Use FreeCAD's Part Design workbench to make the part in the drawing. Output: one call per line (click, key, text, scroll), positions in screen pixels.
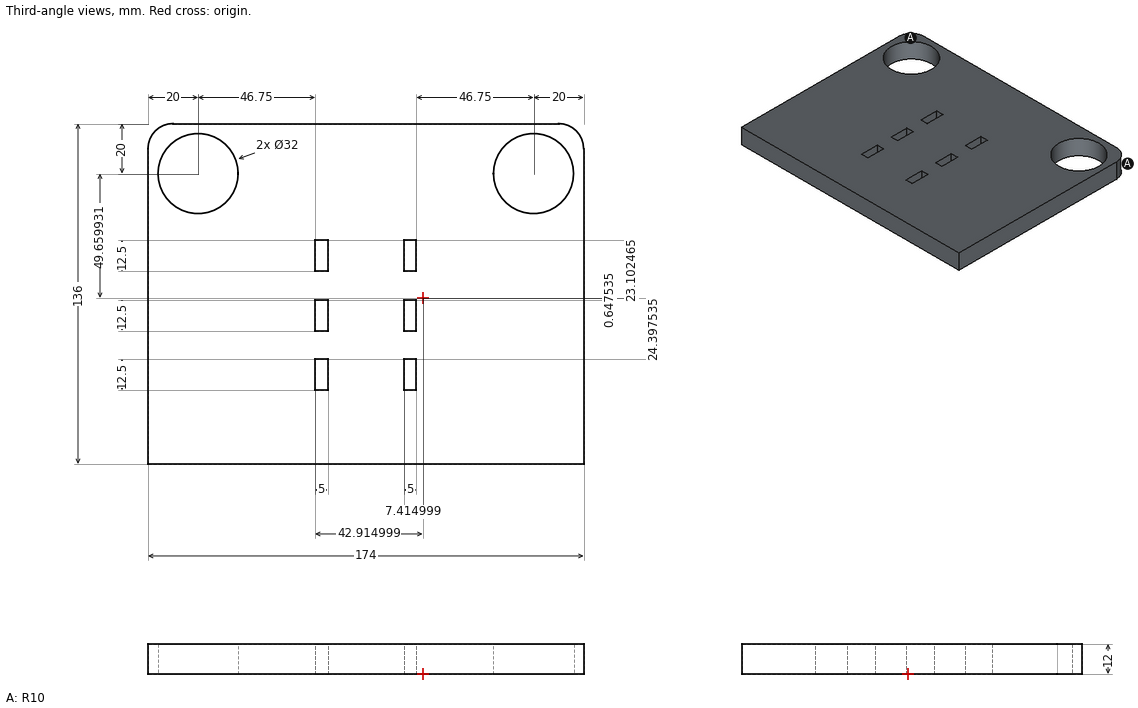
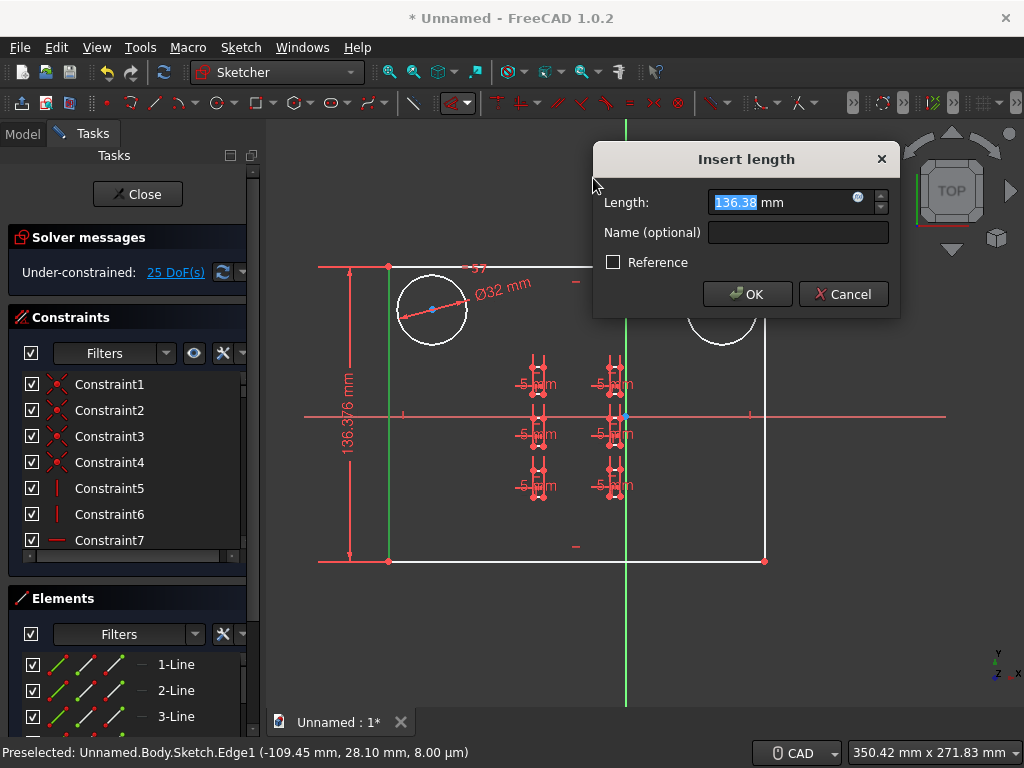
text(136)
key(Return)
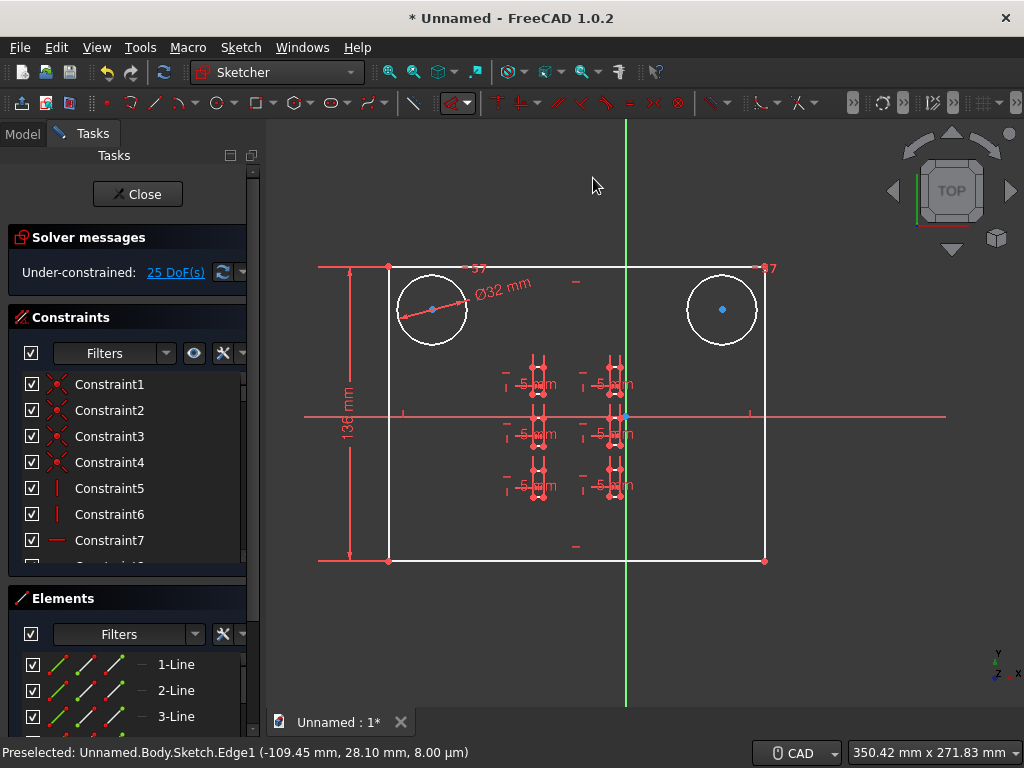
click(502, 561)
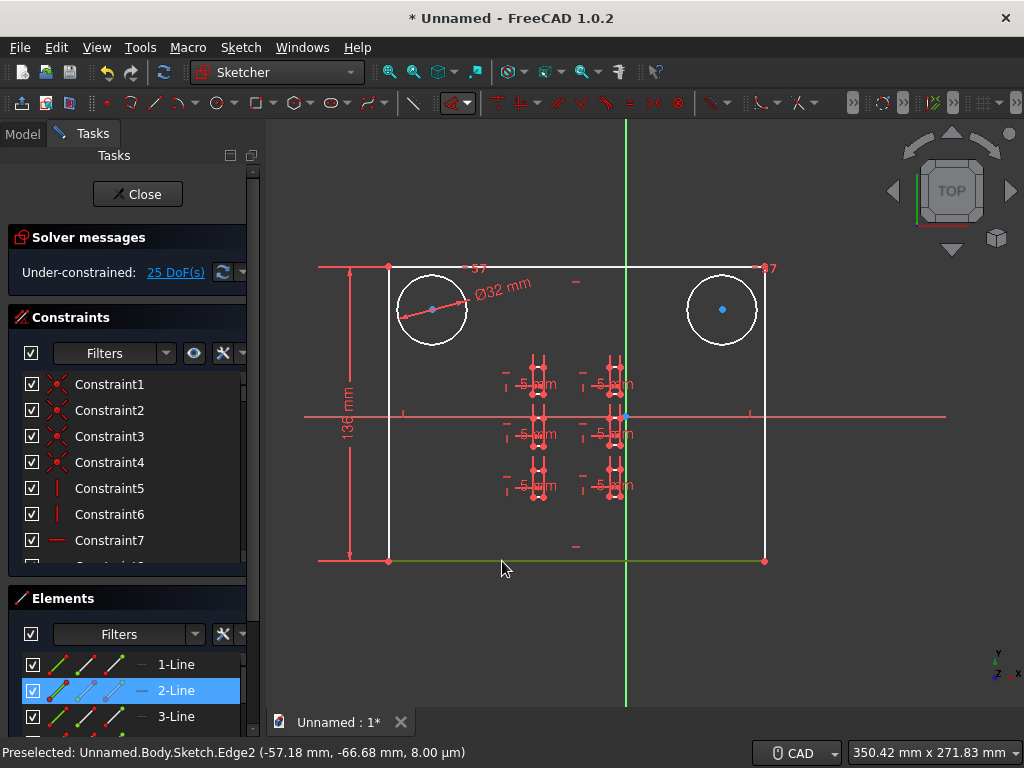
click(470, 104)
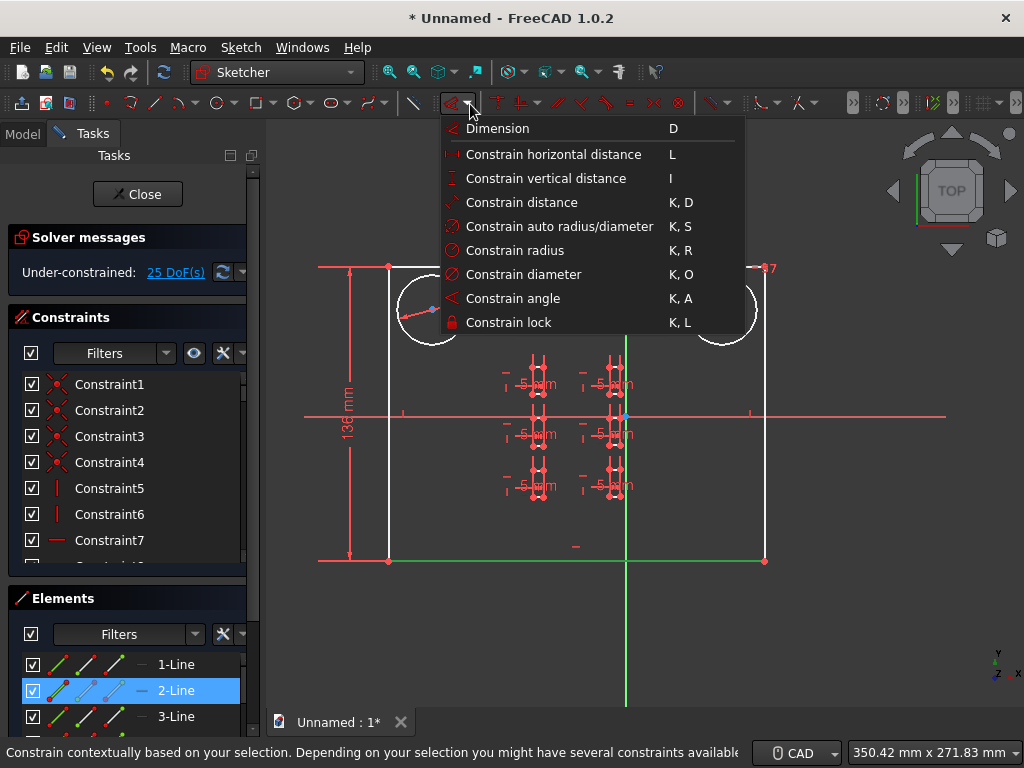
click(593, 154)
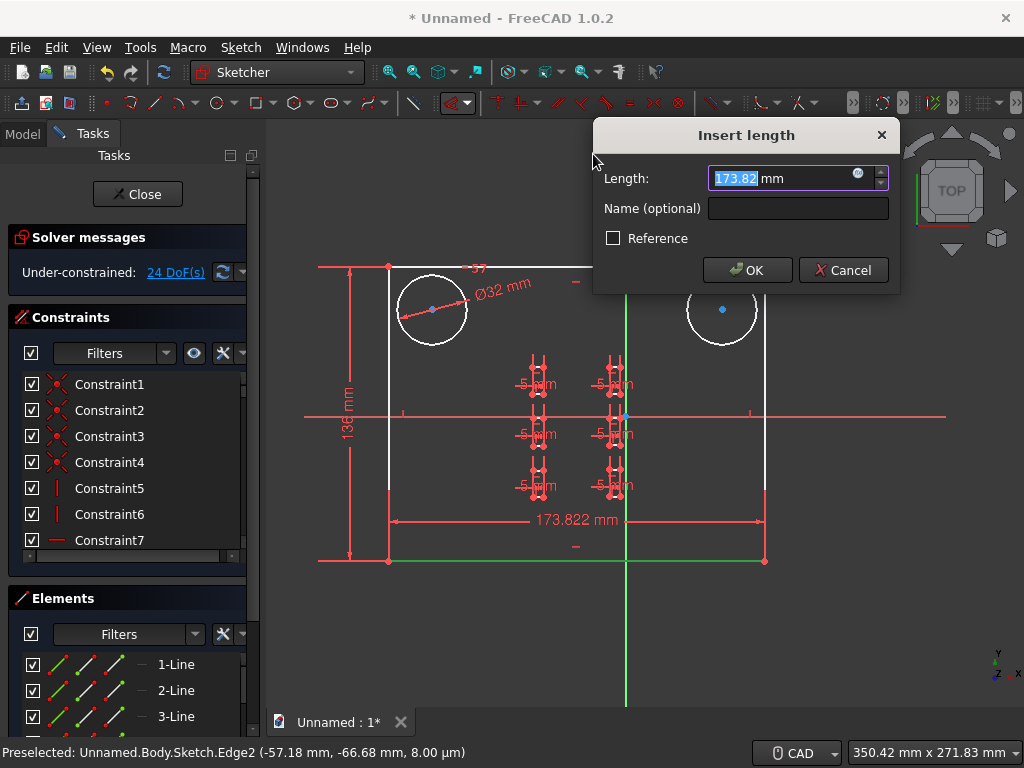
text(174)
key(Return)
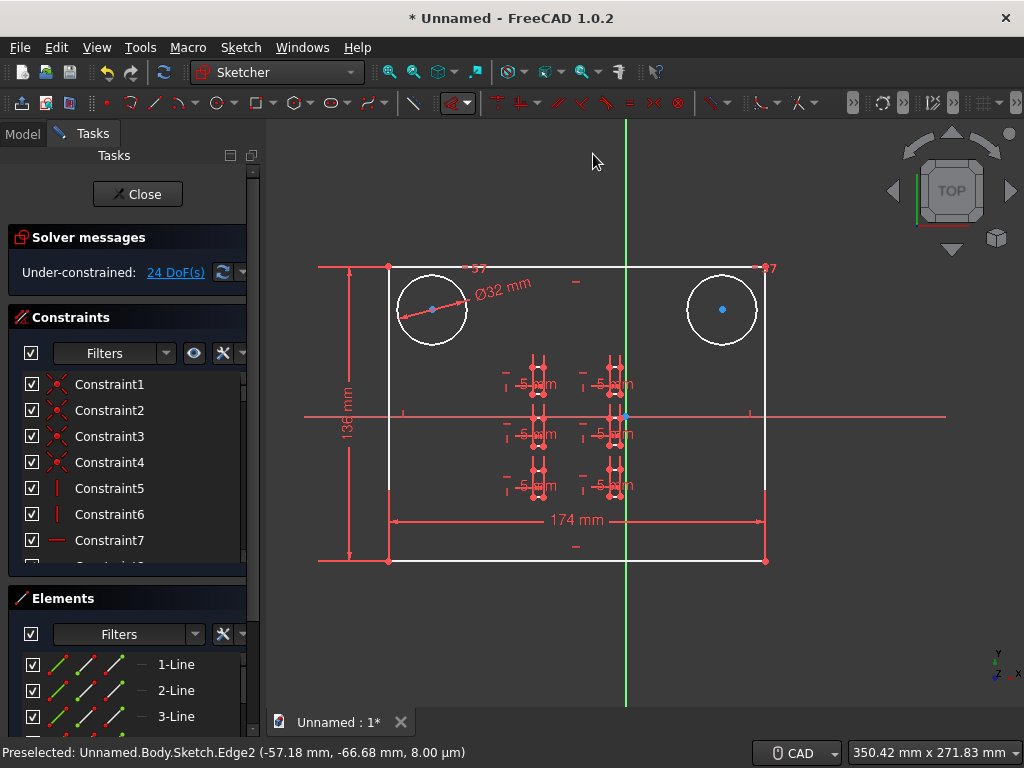
click(389, 267)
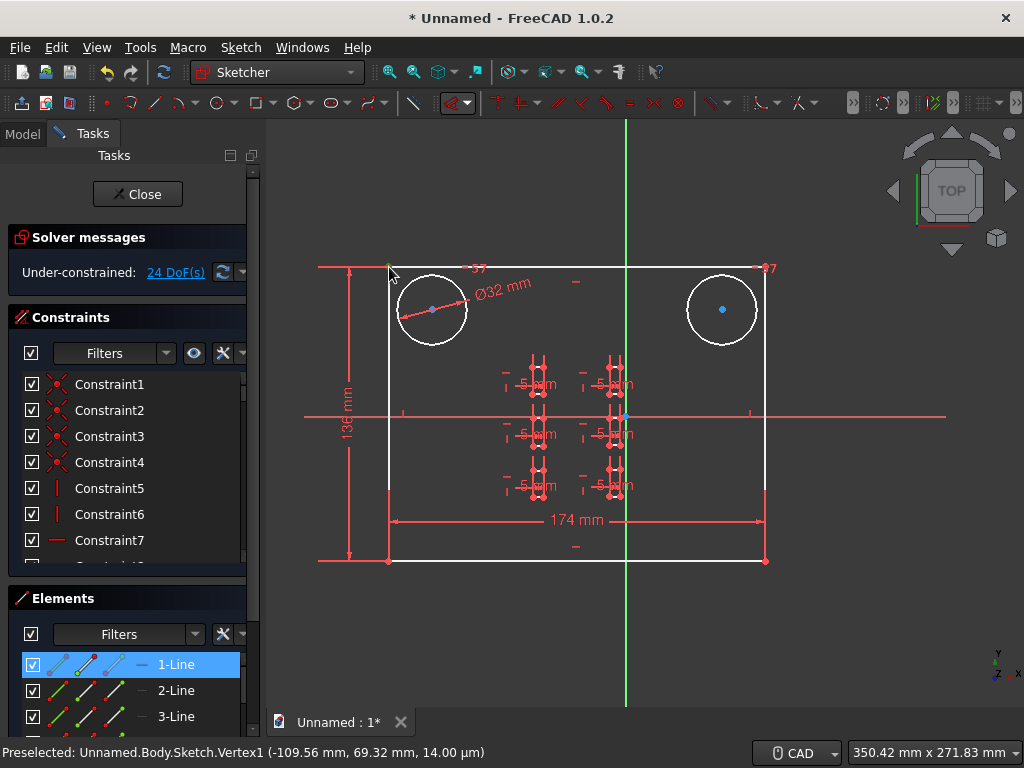
click(432, 310)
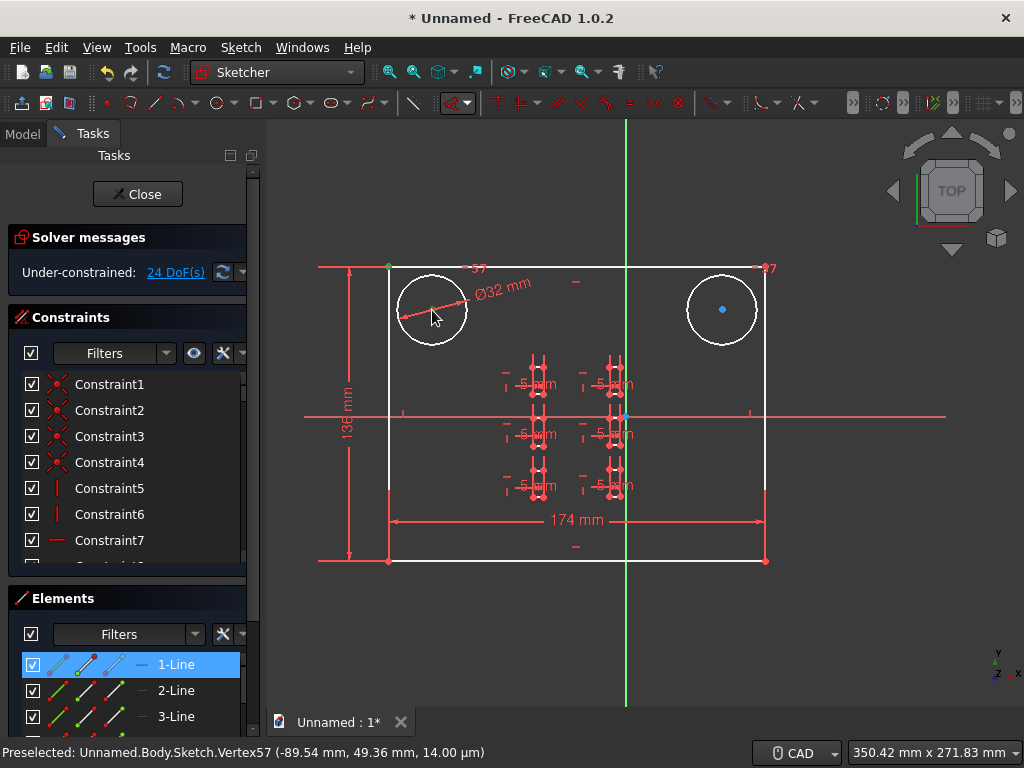
click(470, 104)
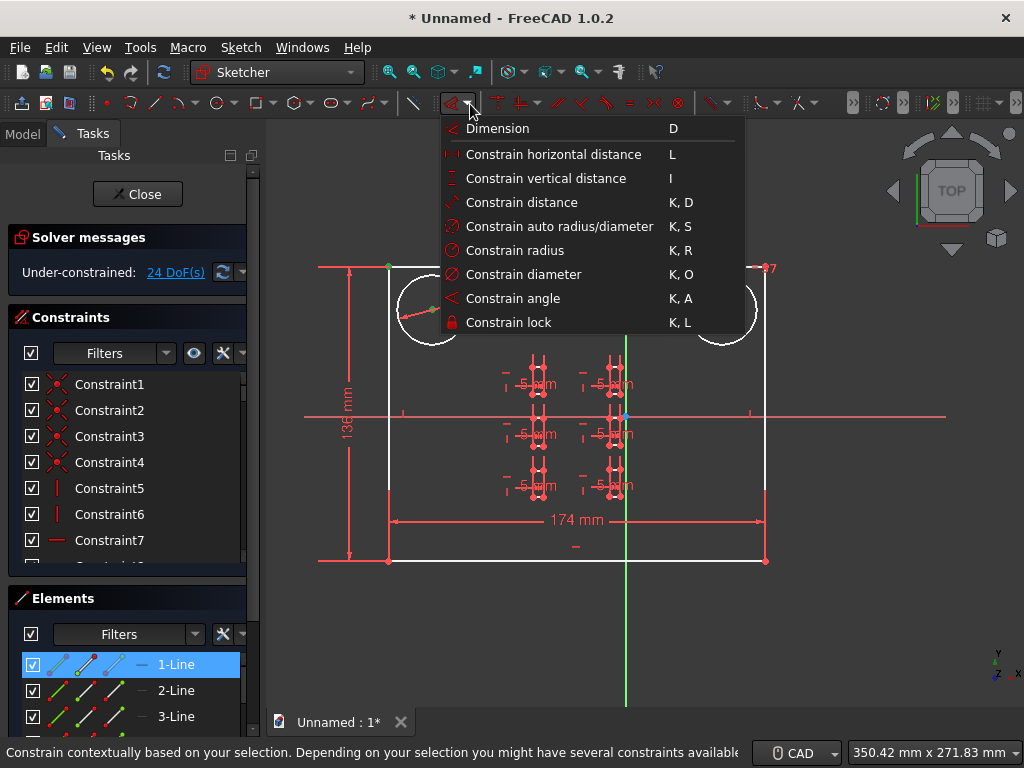
click(593, 154)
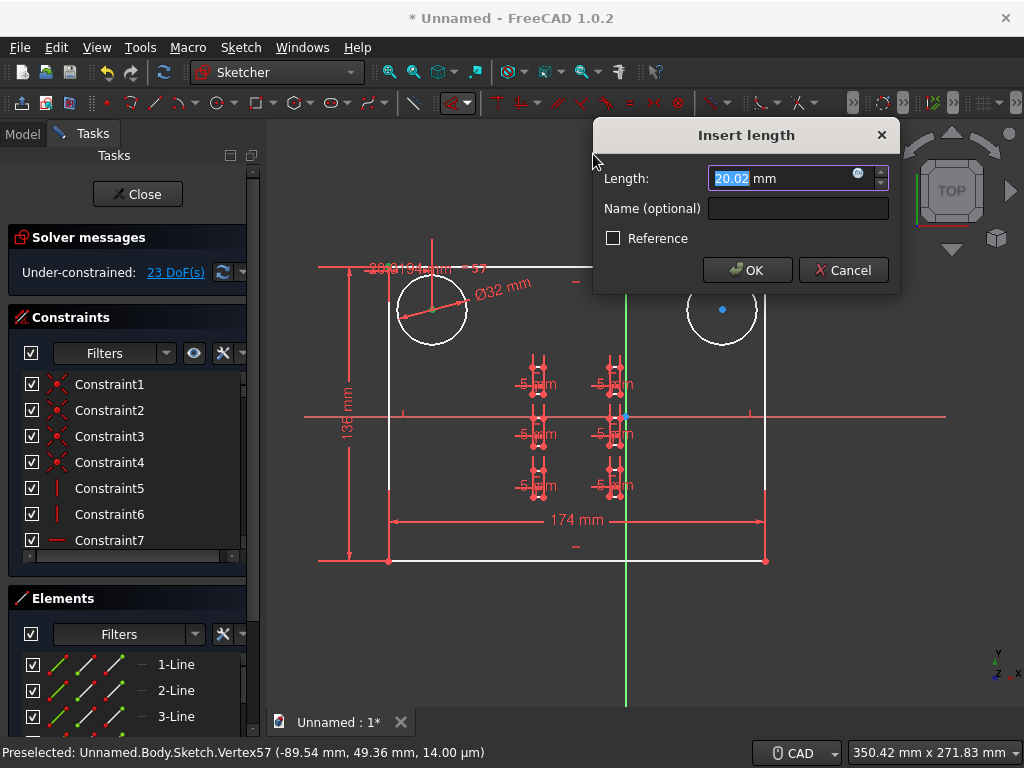
text(20)
key(Return)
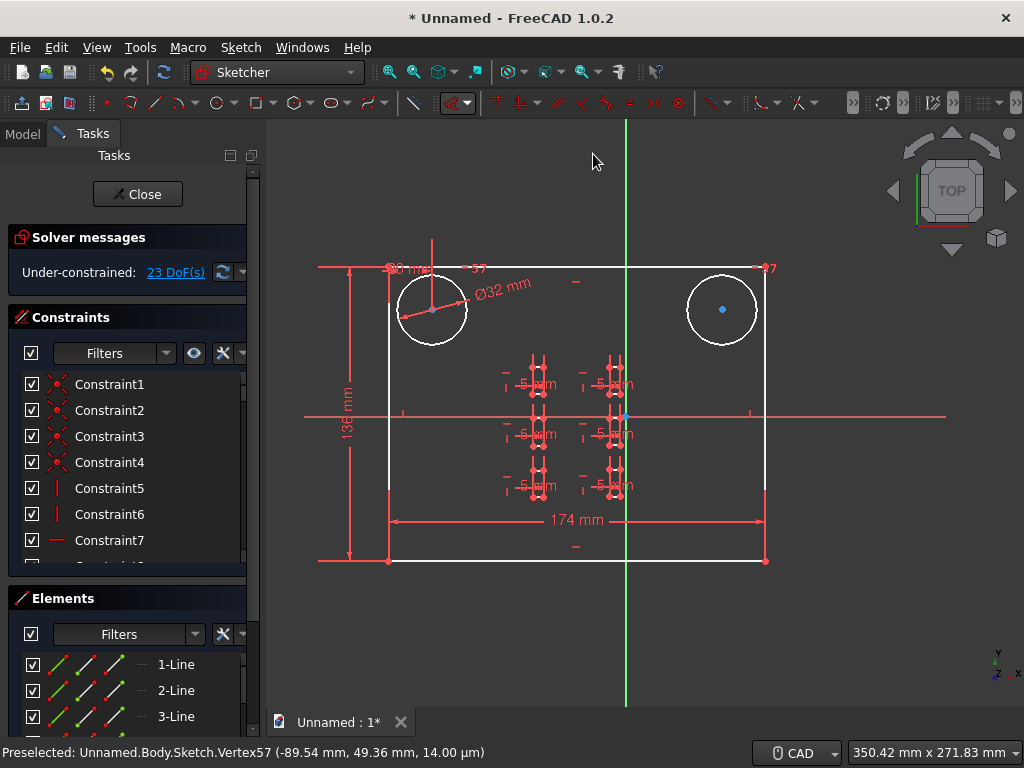
click(389, 267)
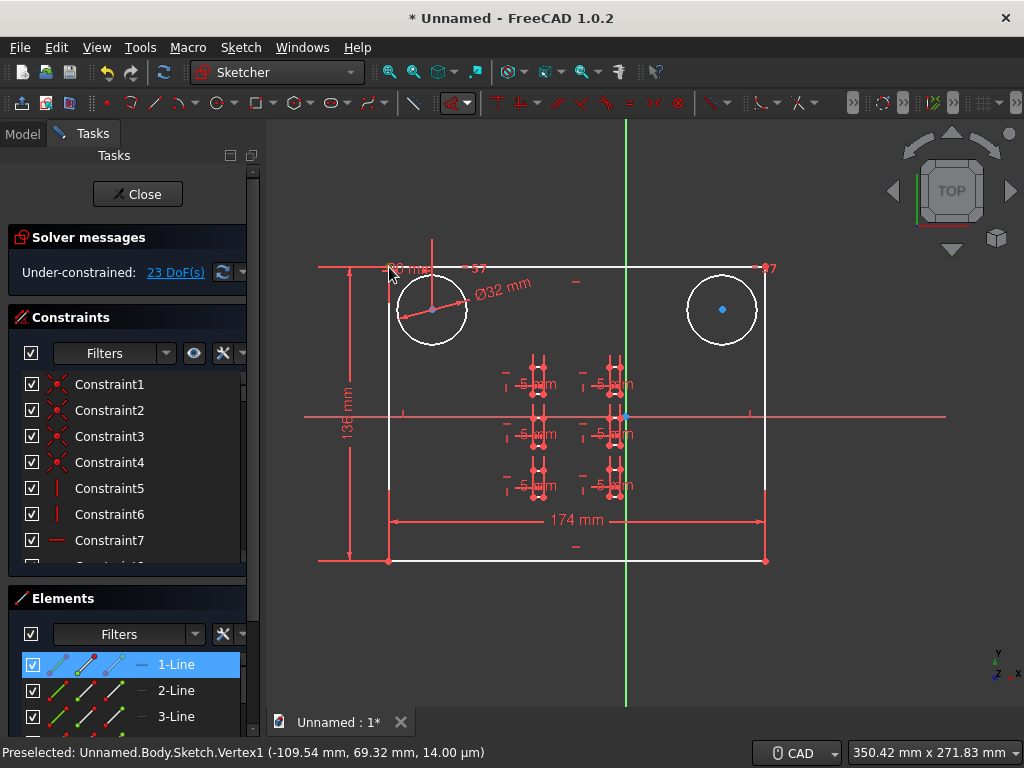
click(432, 310)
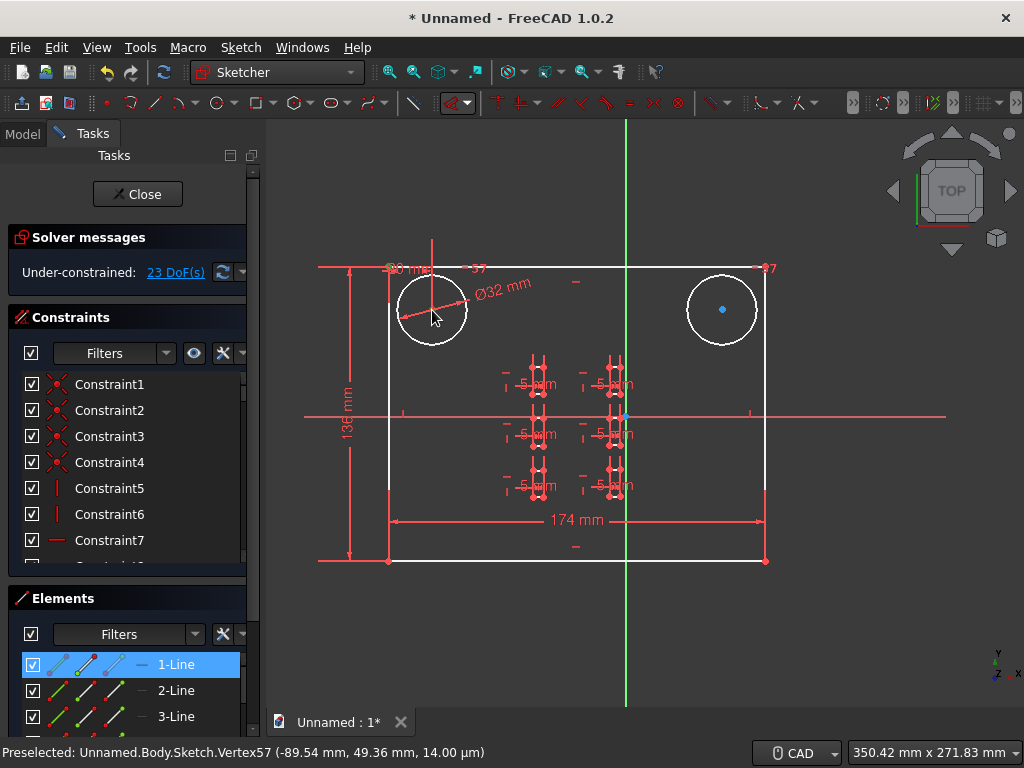
click(470, 104)